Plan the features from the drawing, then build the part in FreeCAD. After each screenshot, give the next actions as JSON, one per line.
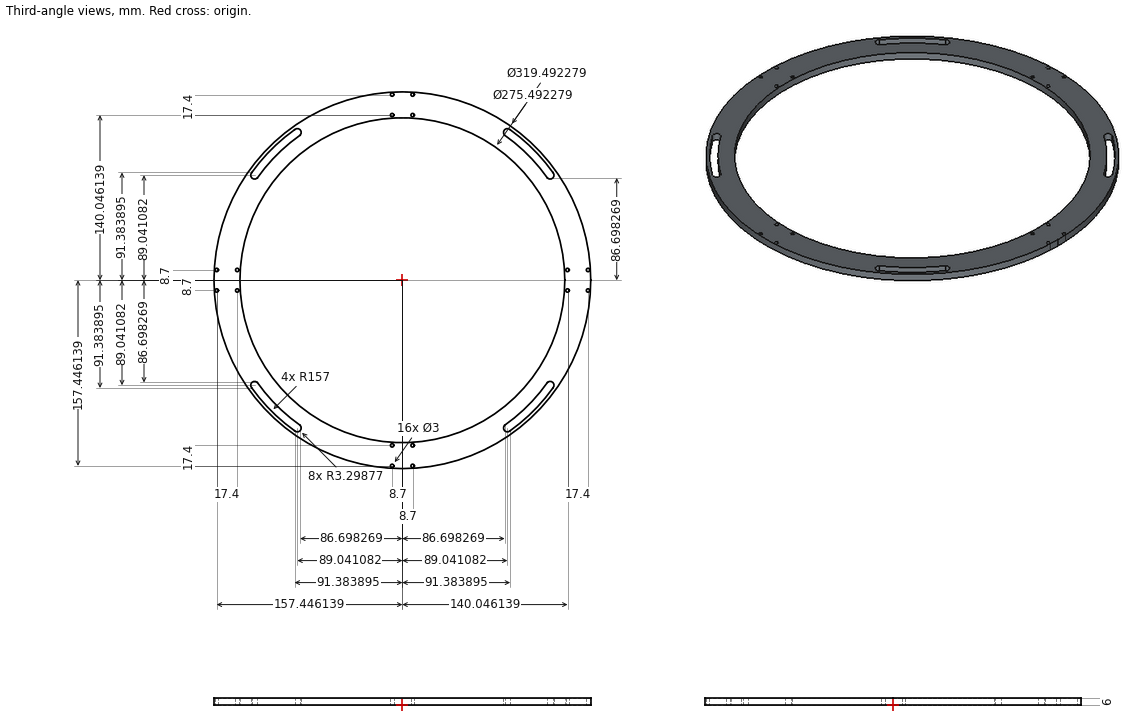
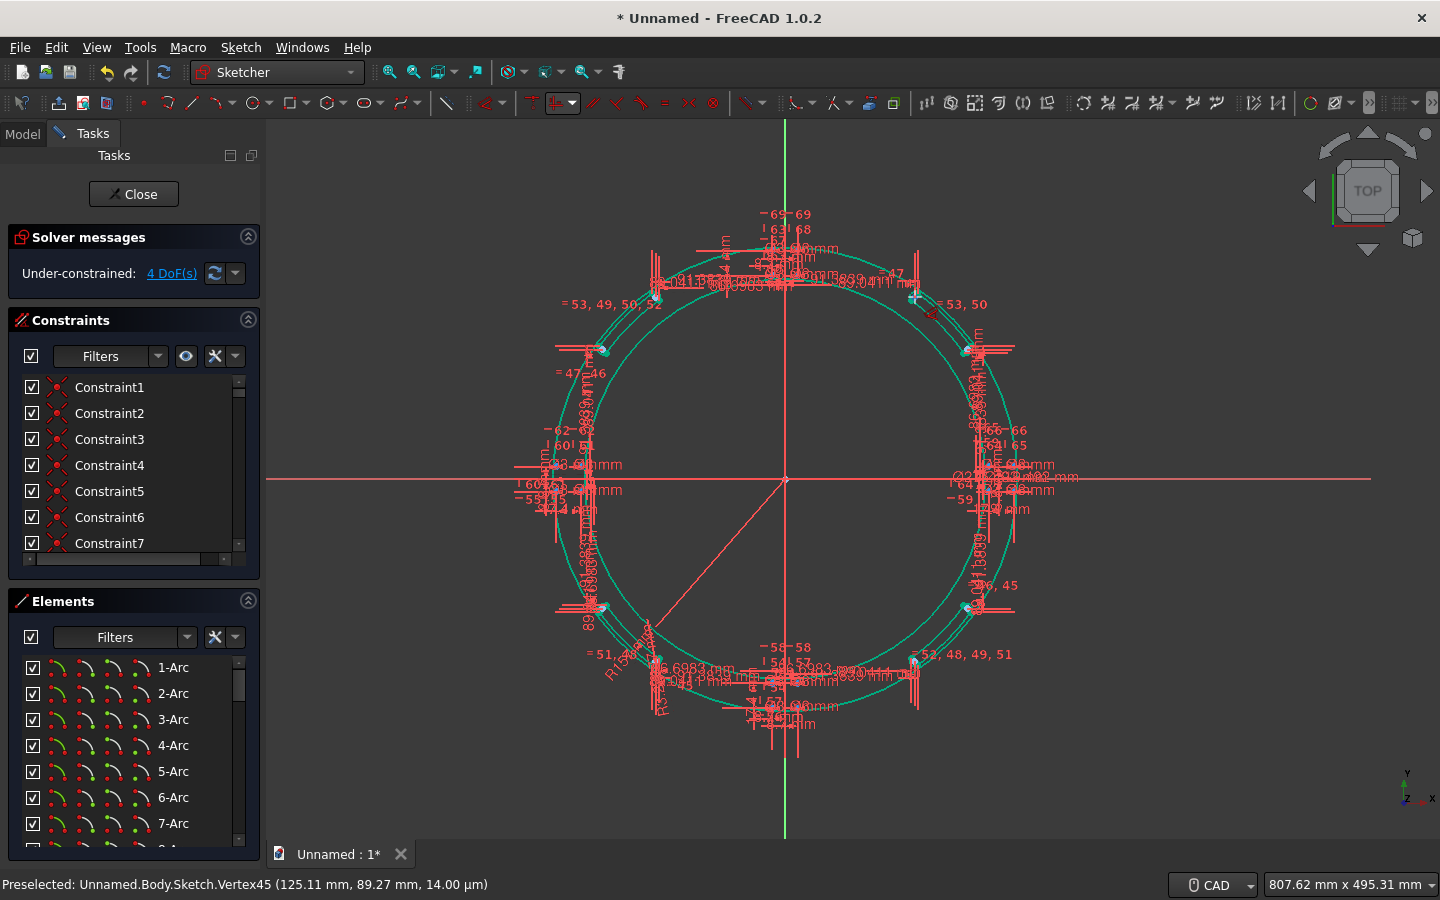
{"action": "left_click", "coordinate": [772, 708]}
{"action": "left_click", "coordinate": [738, 594]}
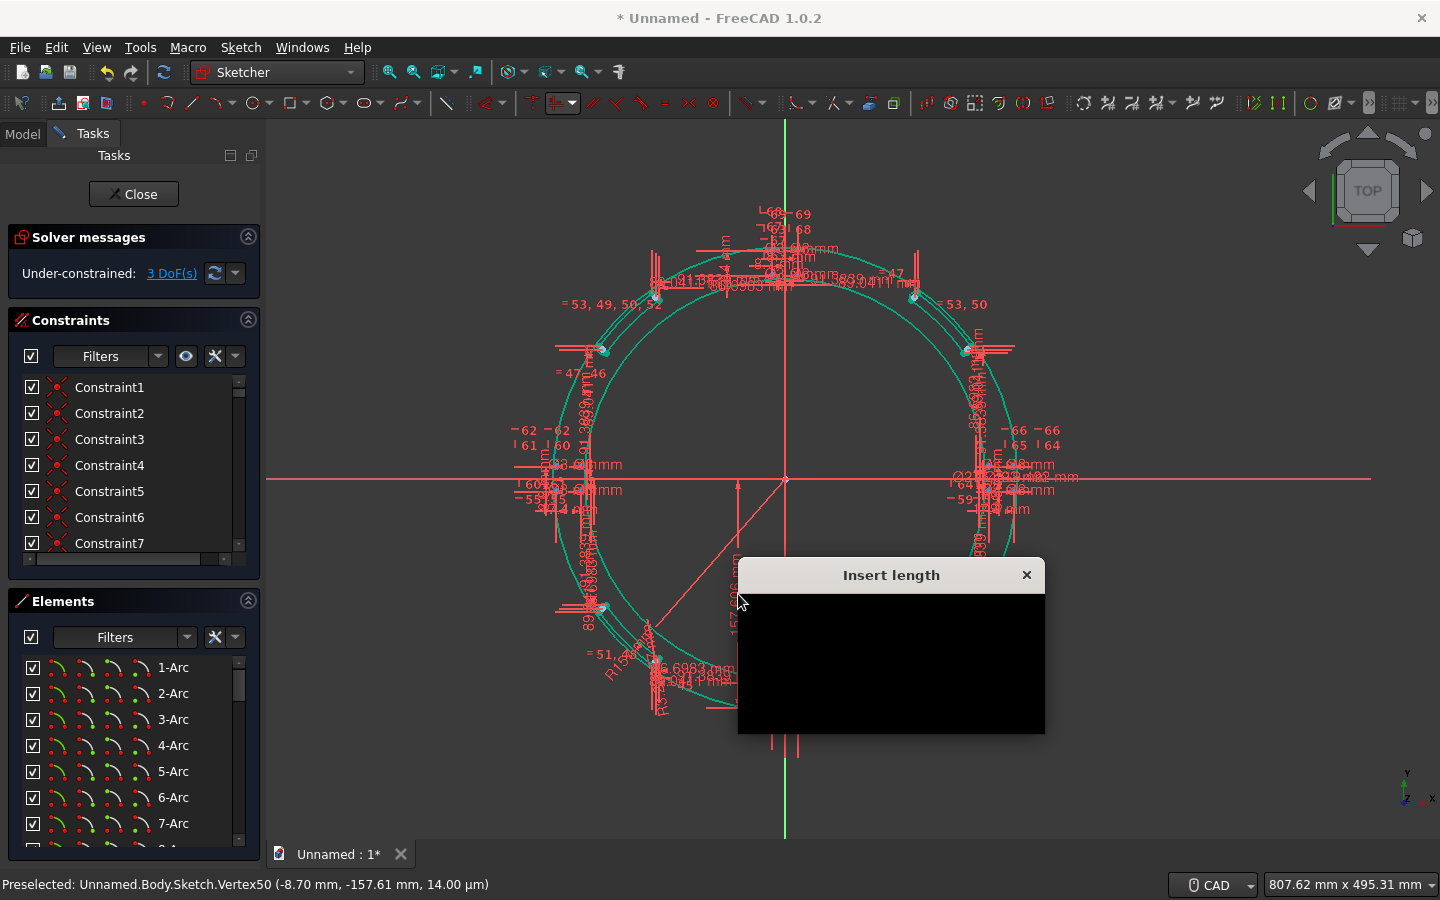
{"action": "type", "text": "157.446139"}
{"action": "key", "text": "Return"}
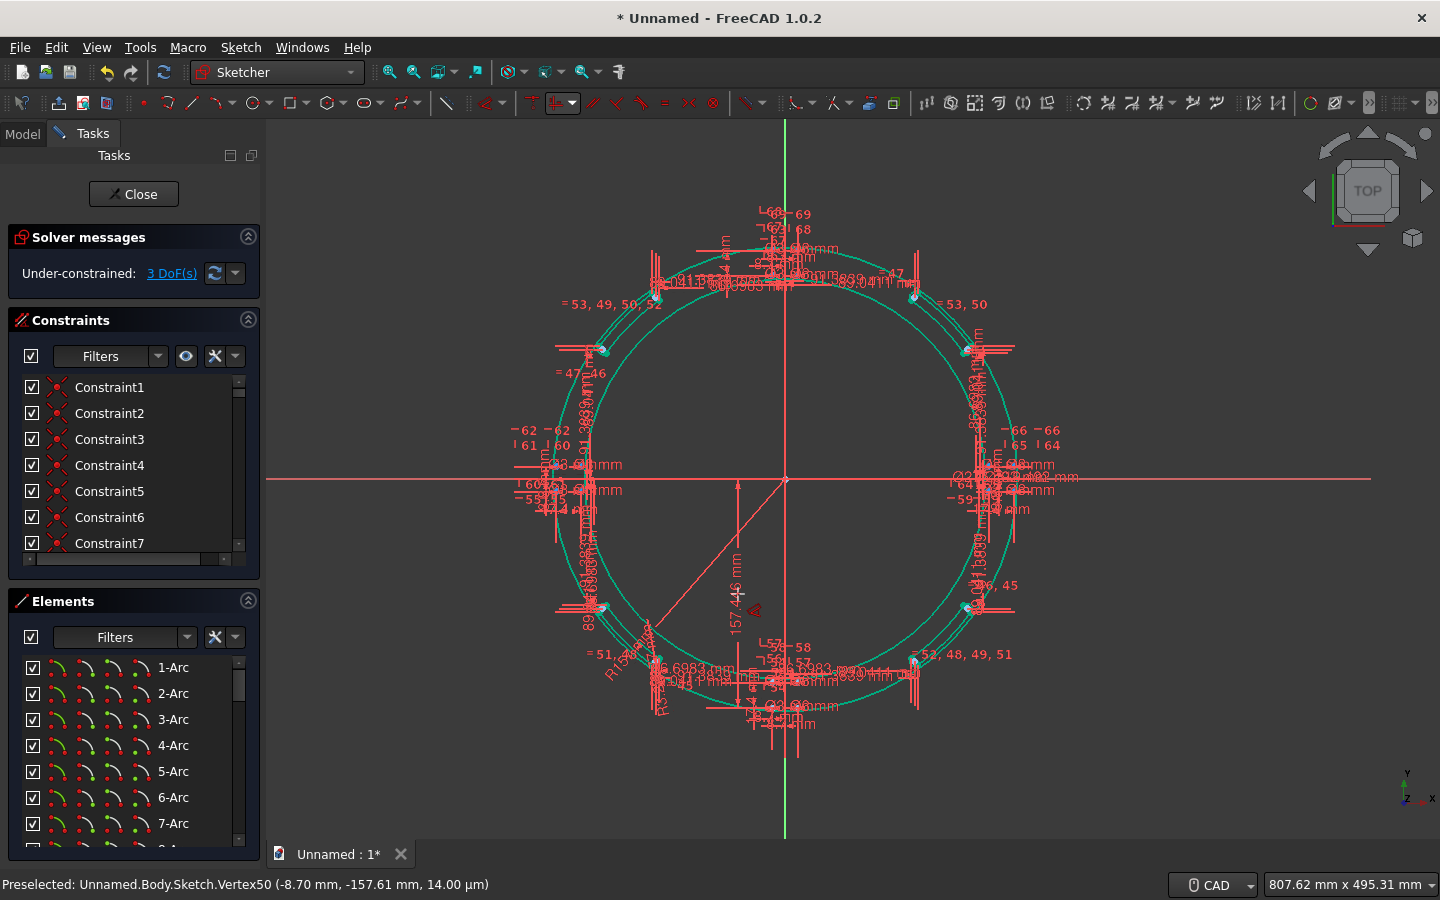
{"action": "left_click", "coordinate": [556, 492]}
{"action": "left_click", "coordinate": [671, 526]}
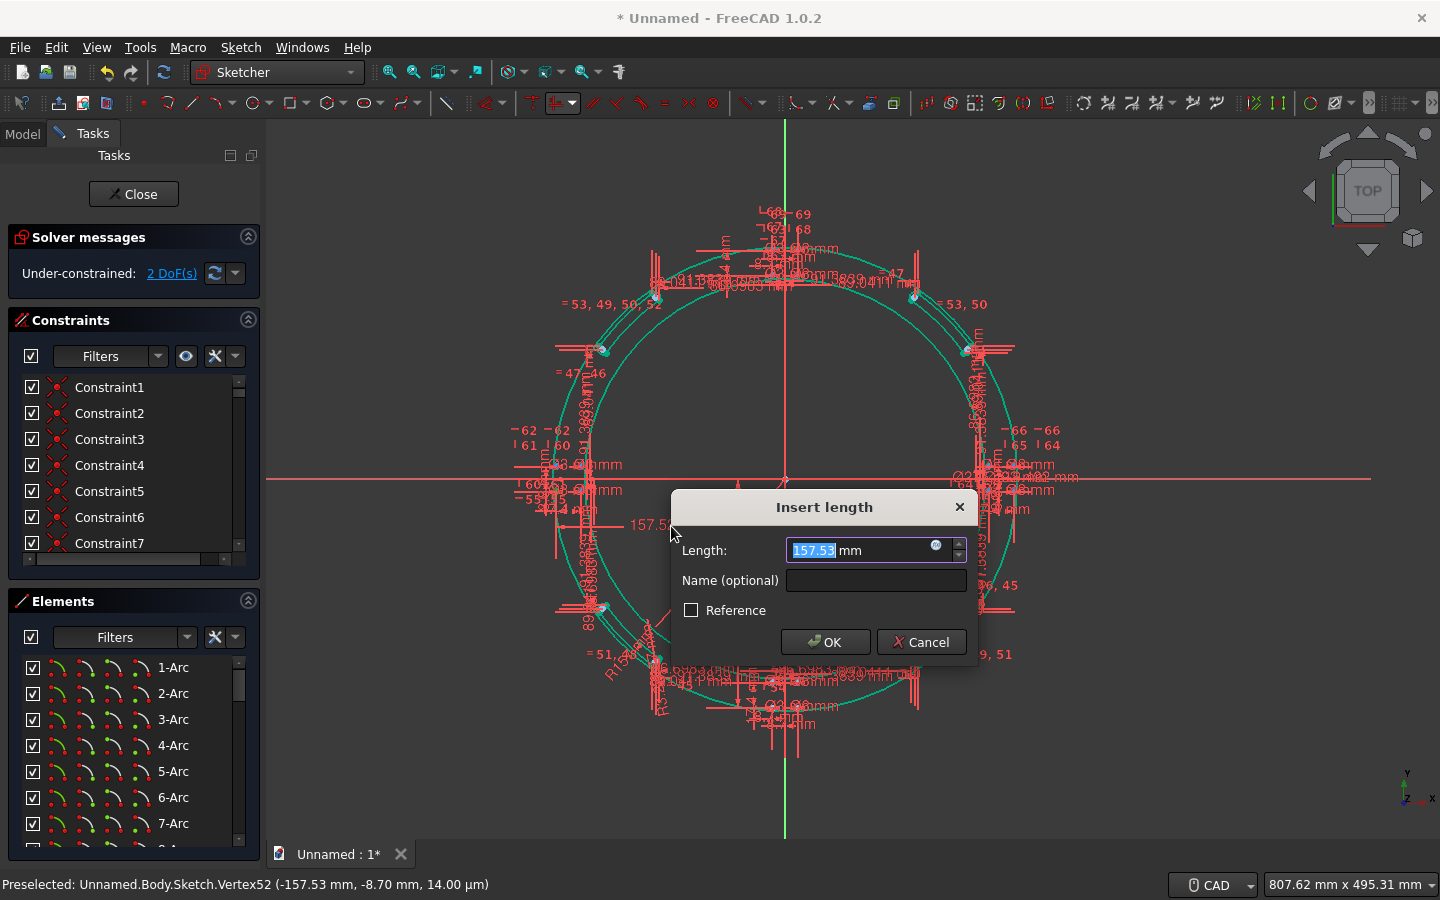
{"action": "type", "text": "157.446139"}
{"action": "key", "text": "Return"}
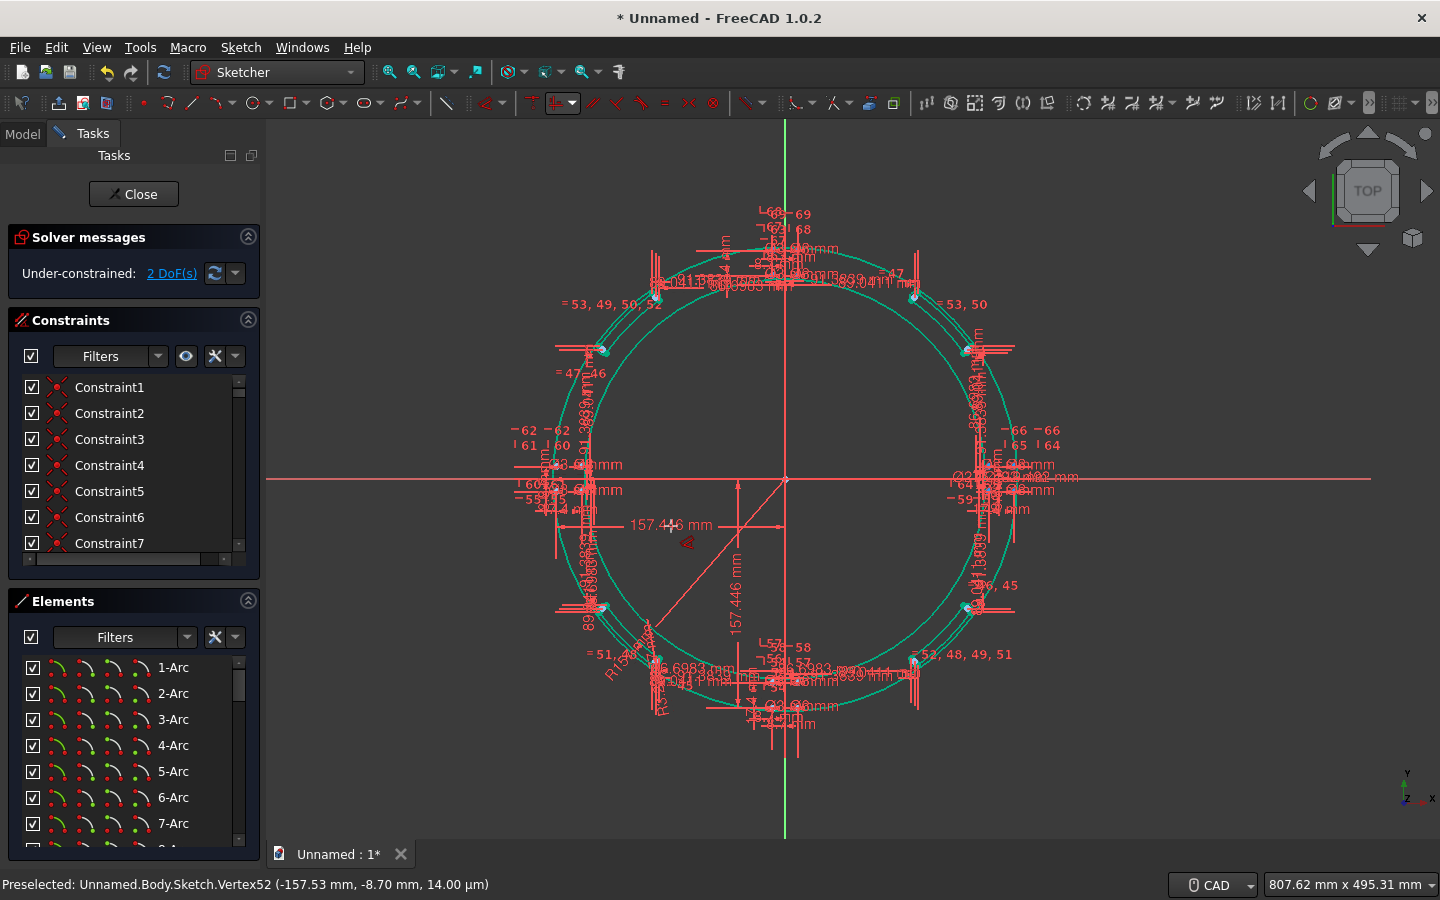
{"action": "left_click", "coordinate": [989, 492]}
{"action": "left_click", "coordinate": [887, 526]}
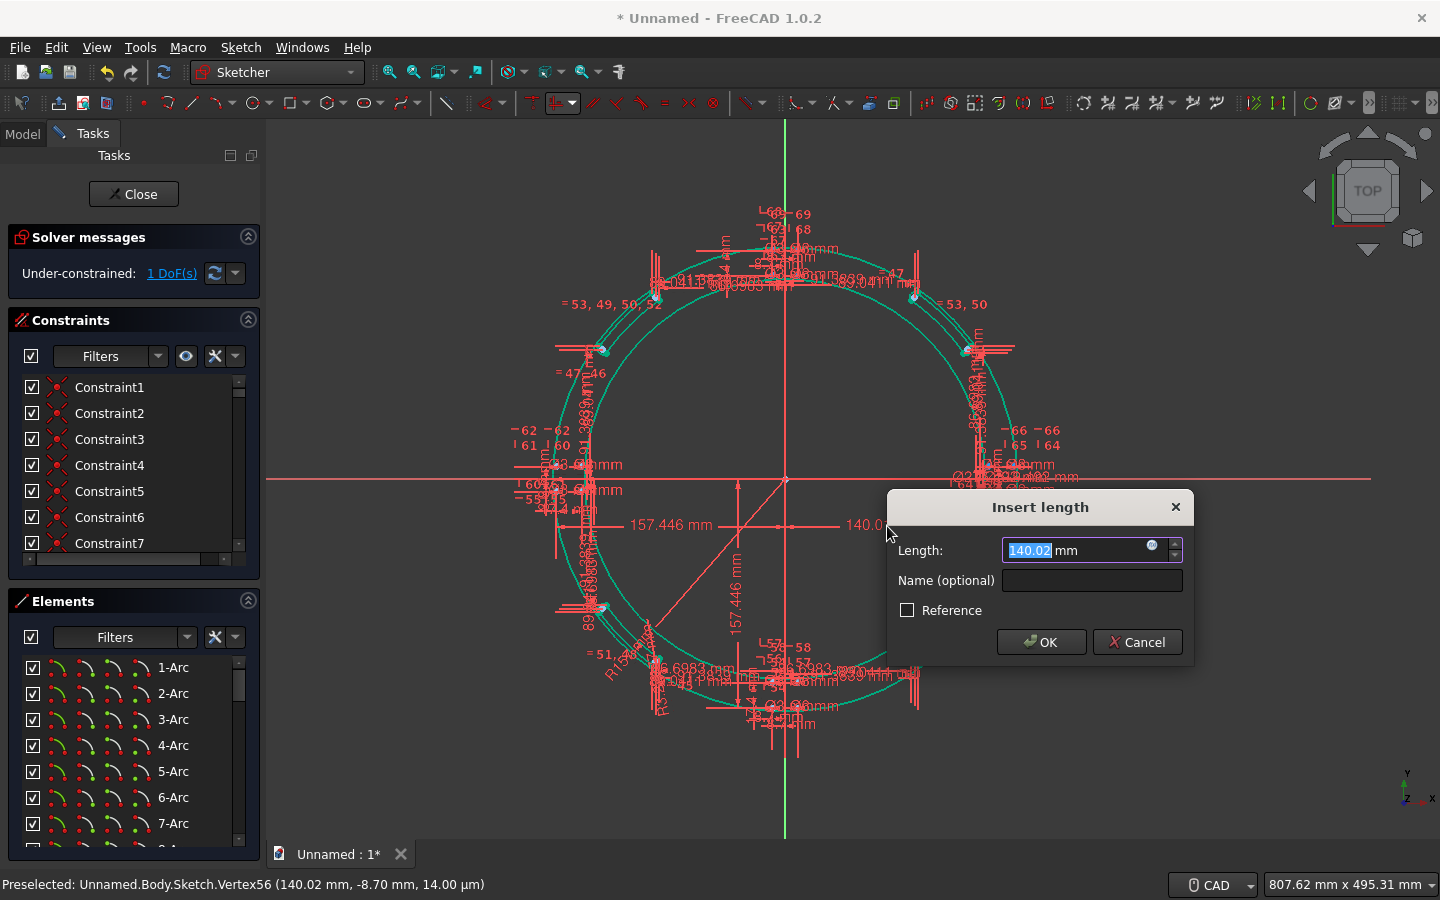
{"action": "type", "text": "140.046139"}
{"action": "key", "text": "Return"}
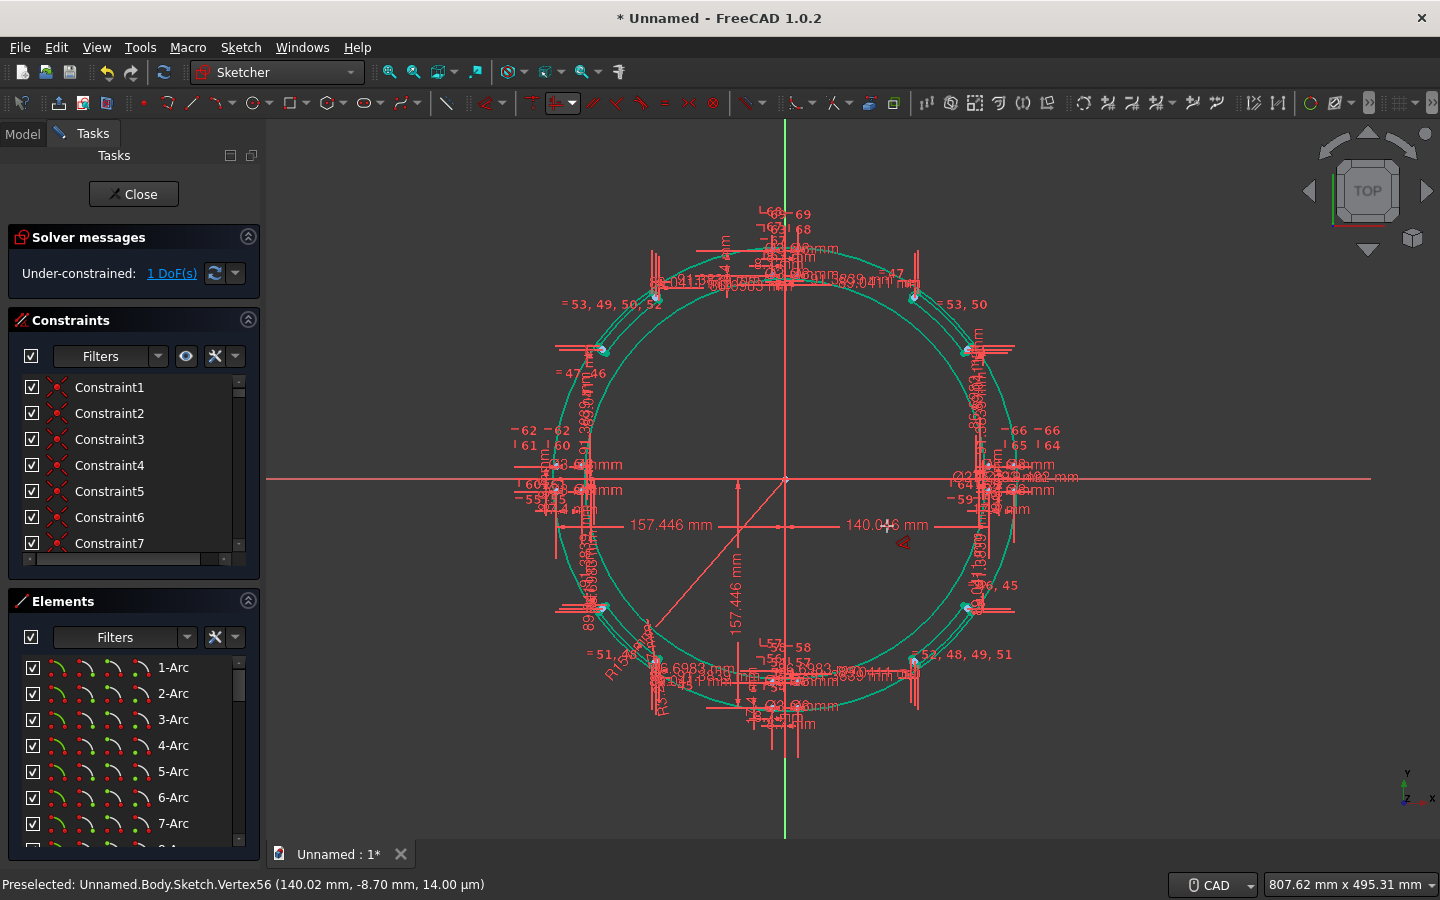
{"action": "left_click", "coordinate": [772, 276]}
{"action": "left_click", "coordinate": [738, 378]}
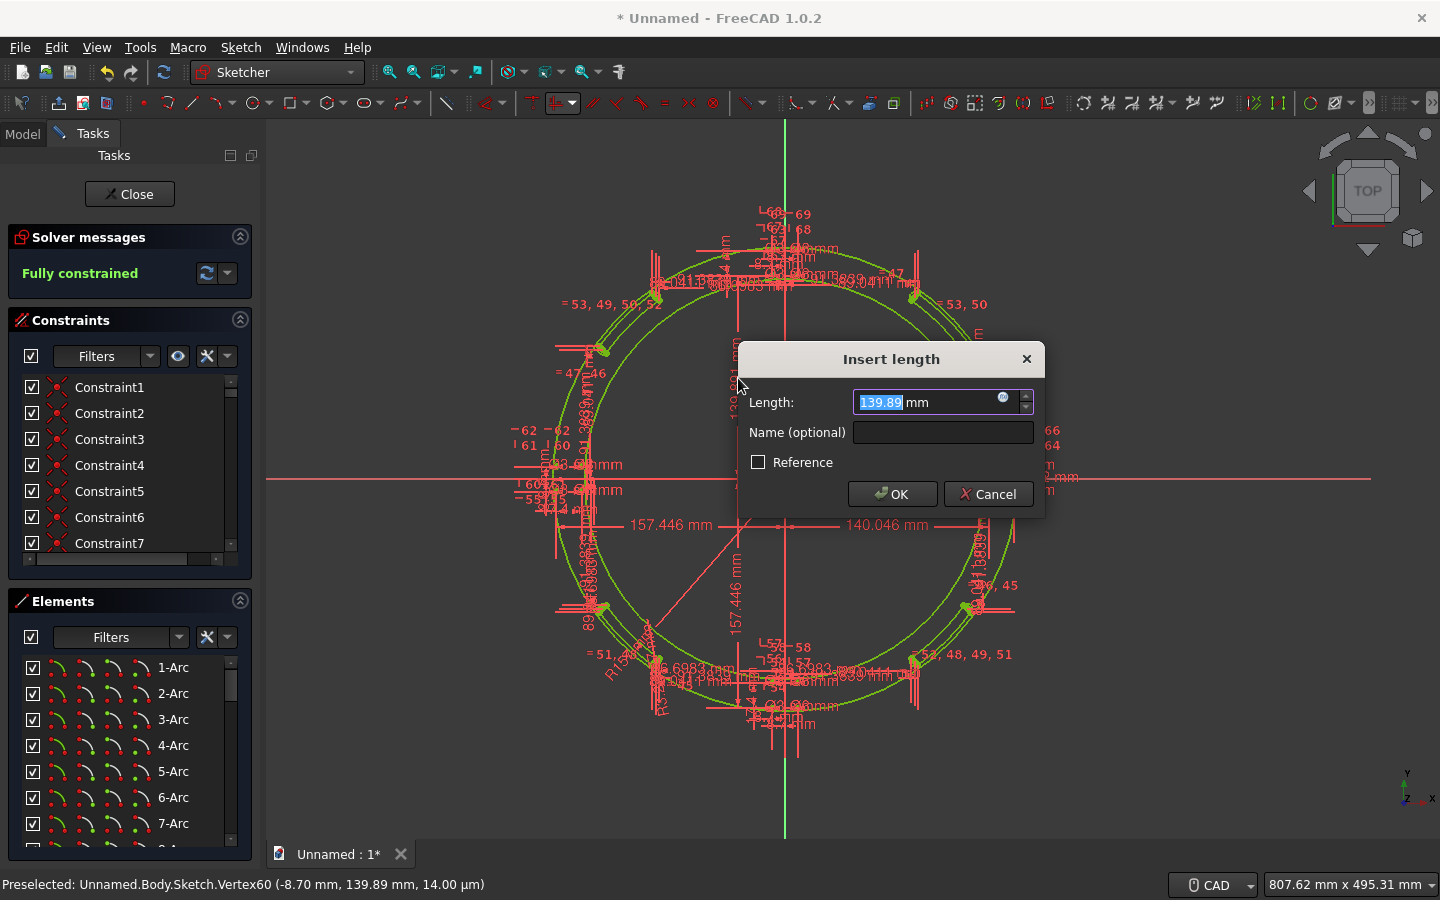
{"action": "type", "text": "140.046139"}
{"action": "key", "text": "Return"}
{"action": "key", "text": "Escape"}